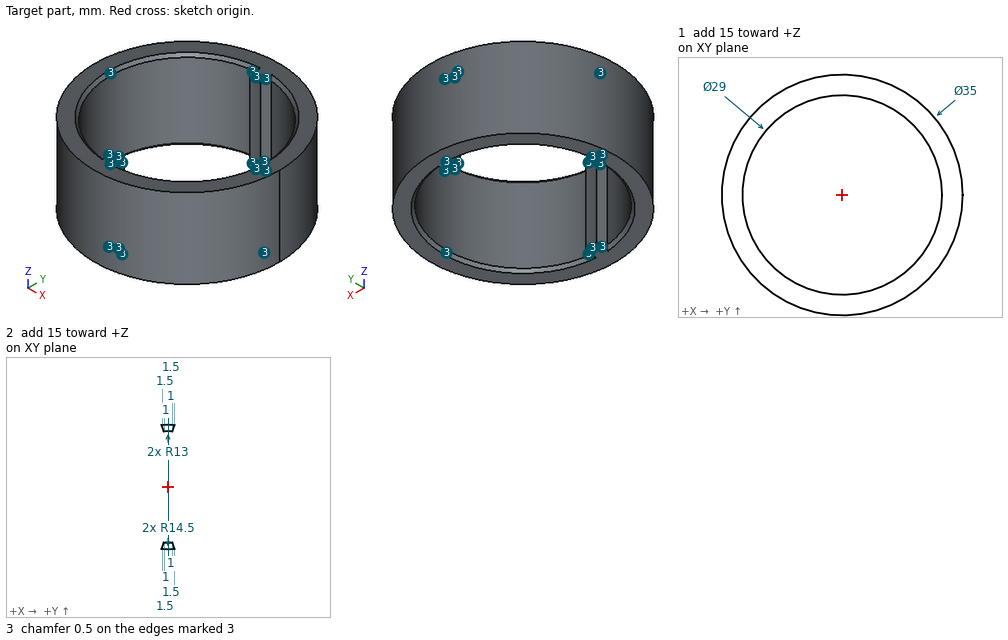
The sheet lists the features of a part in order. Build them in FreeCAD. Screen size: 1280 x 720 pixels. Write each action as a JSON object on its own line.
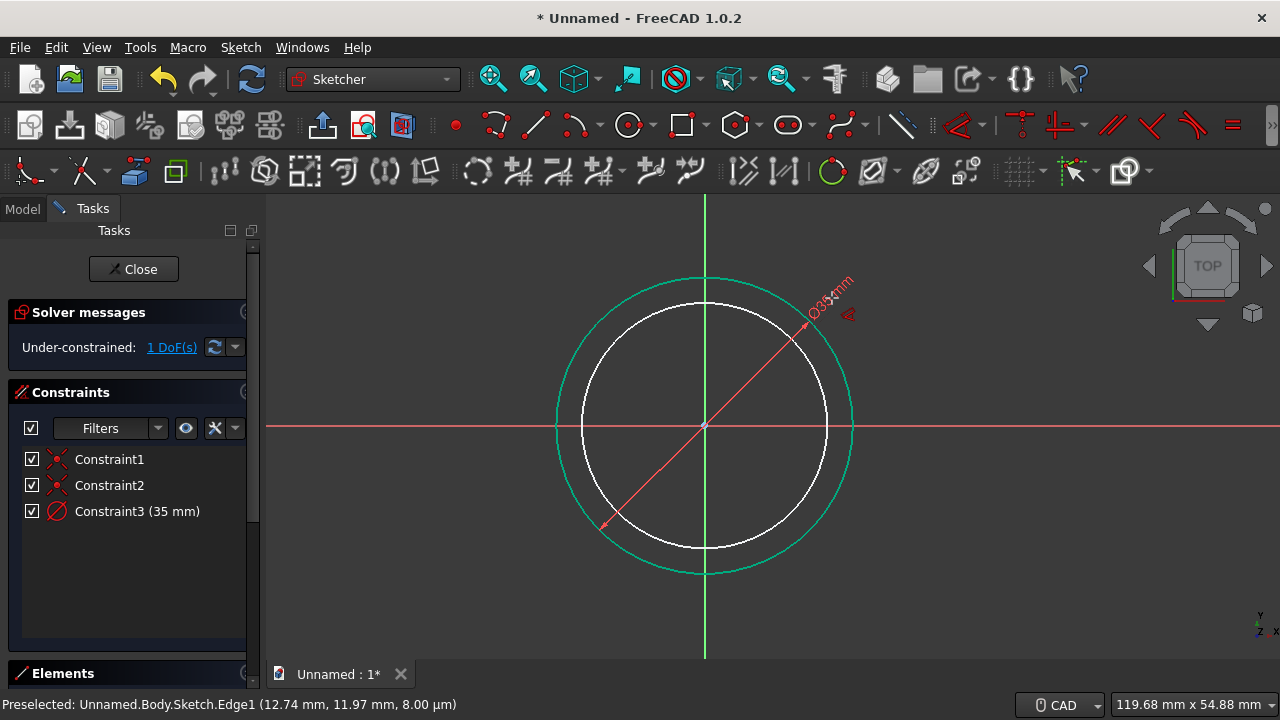
{"action": "left_click", "coordinate": [791, 339]}
{"action": "left_click", "coordinate": [875, 375]}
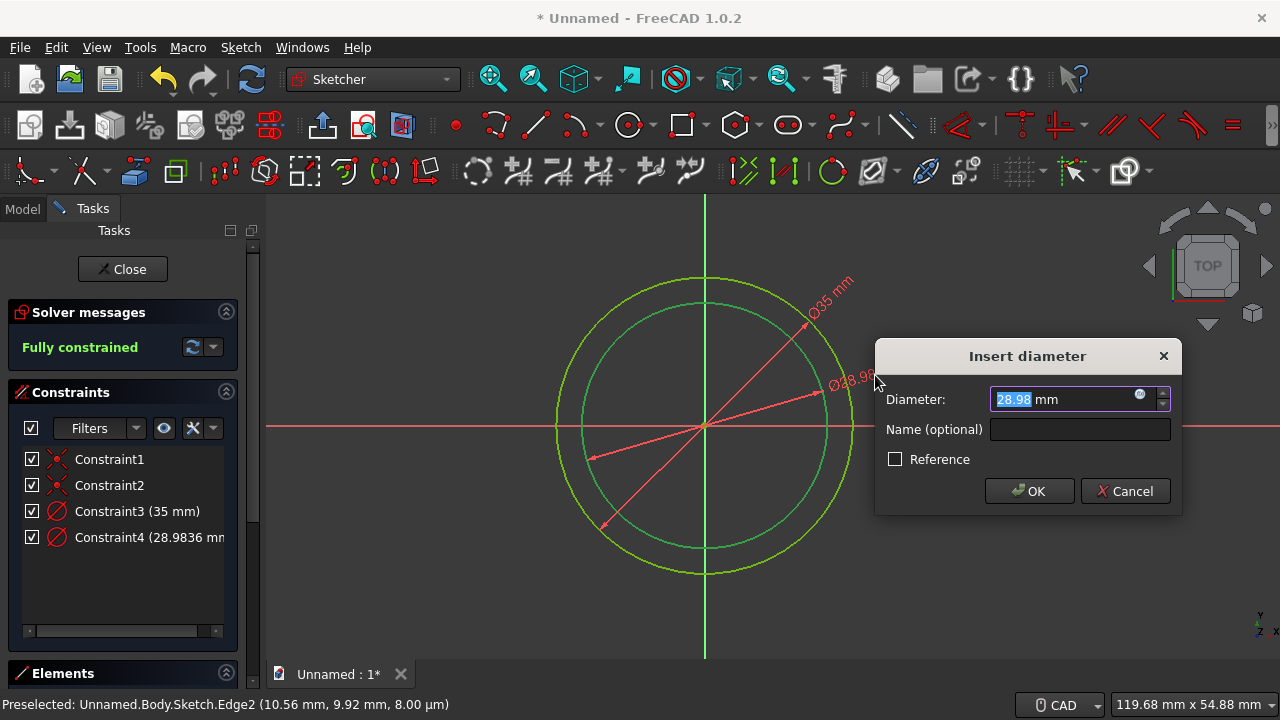
{"action": "type", "text": "29"}
{"action": "key", "text": "Return"}
{"action": "key", "text": "Escape"}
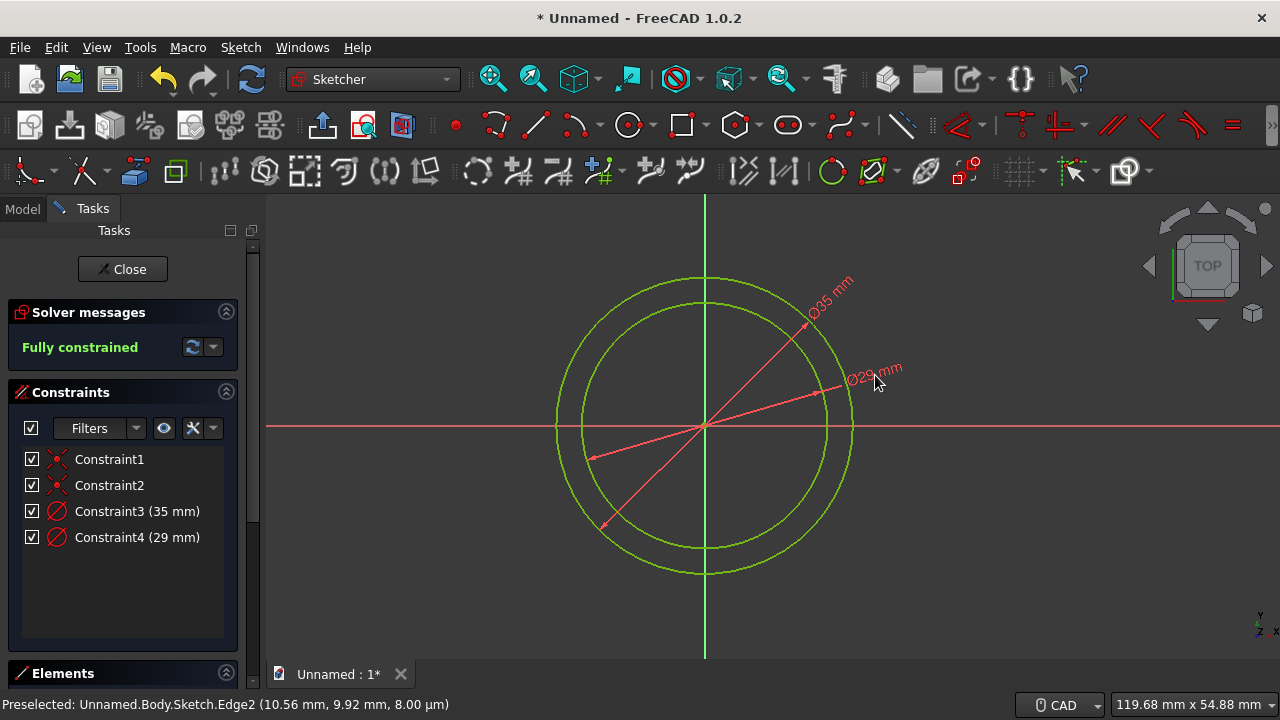
{"action": "left_click", "coordinate": [123, 269]}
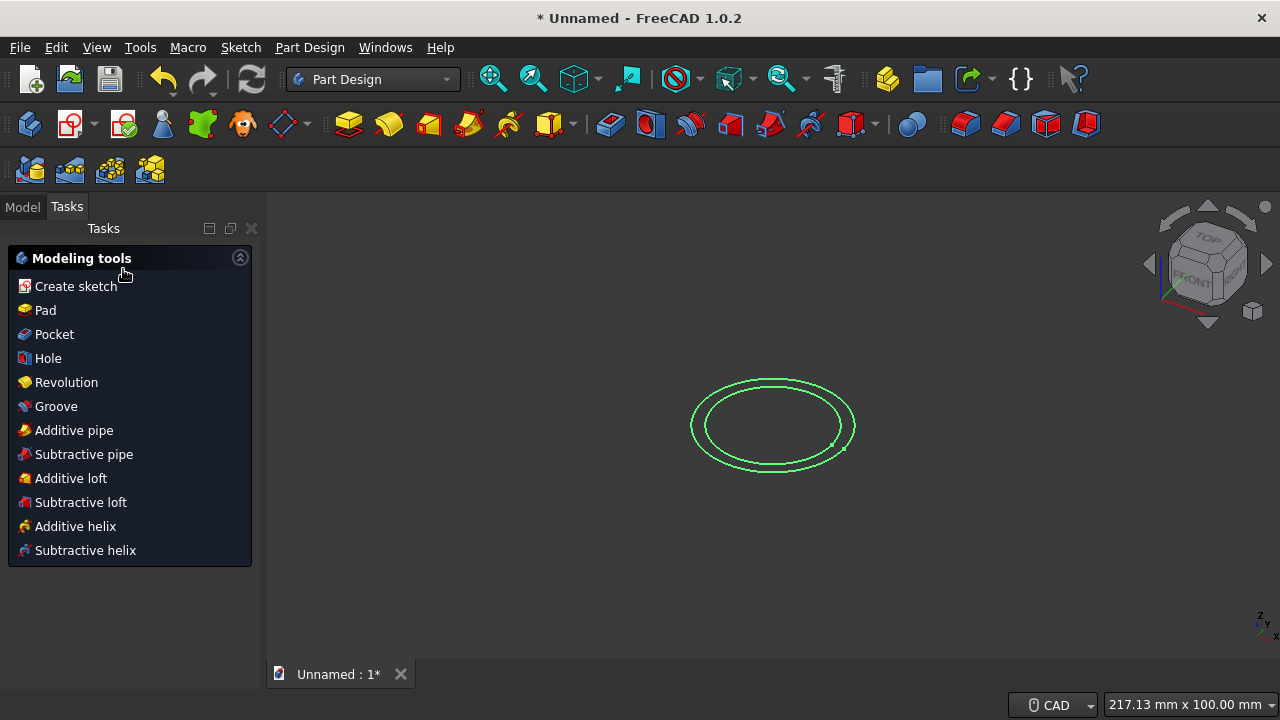
{"action": "left_click", "coordinate": [350, 124]}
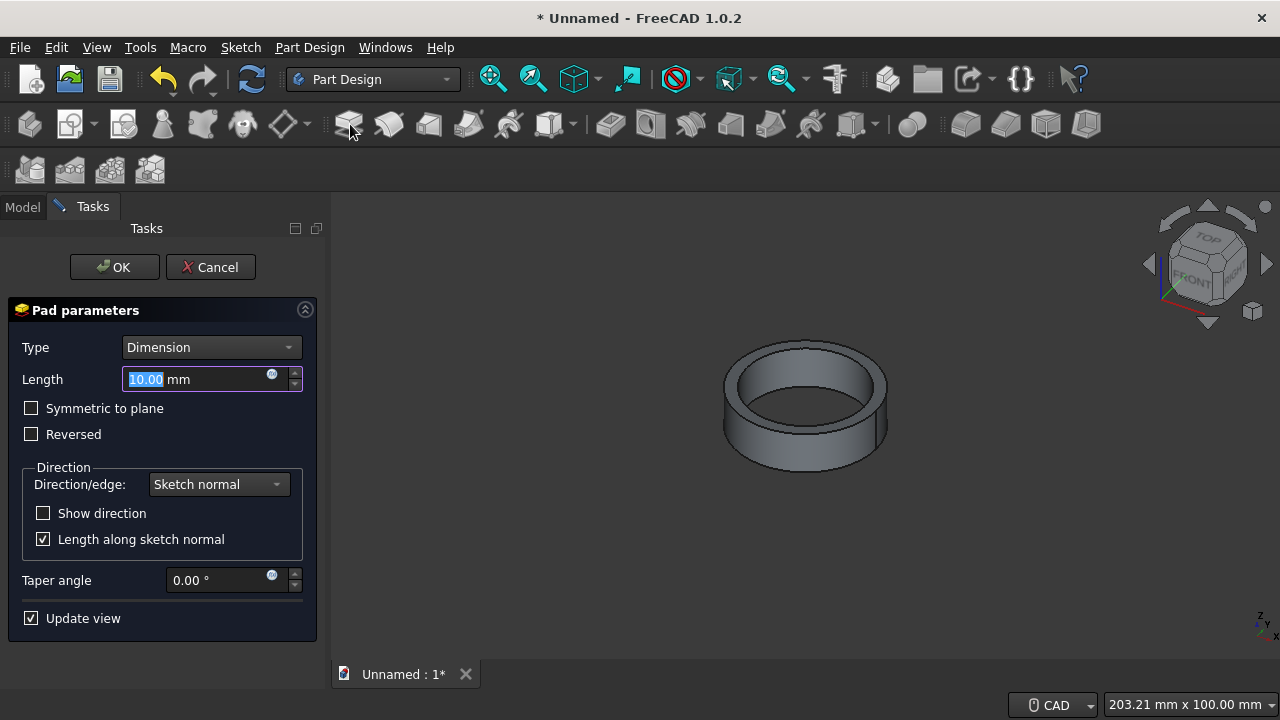
{"action": "type", "text": "15"}
{"action": "key", "text": "Tab"}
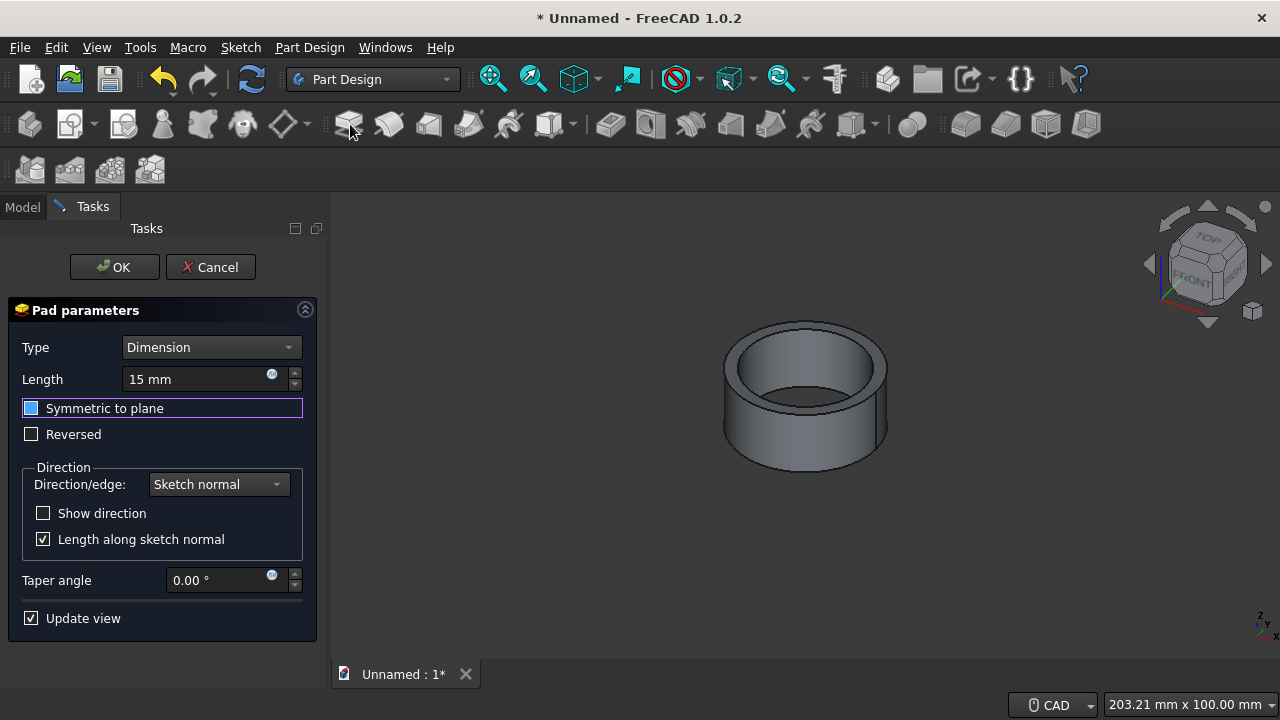
{"action": "left_click", "coordinate": [115, 267]}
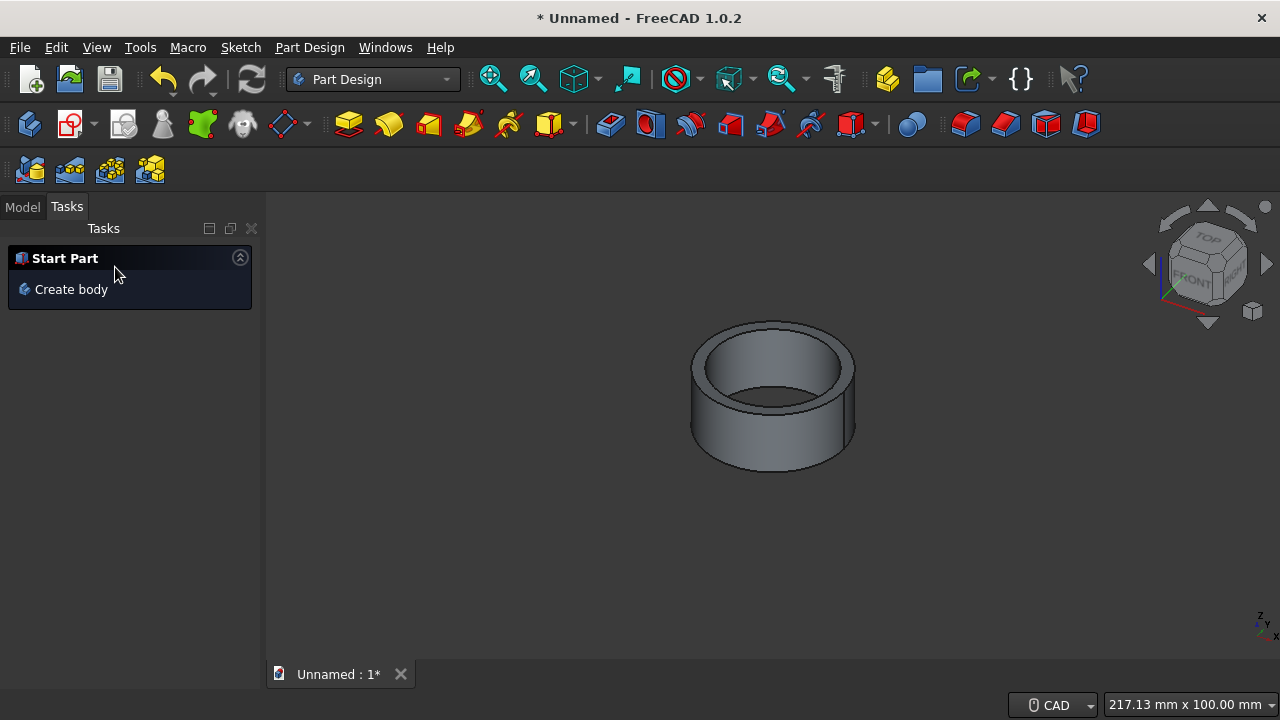
{"action": "key", "text": "v f"}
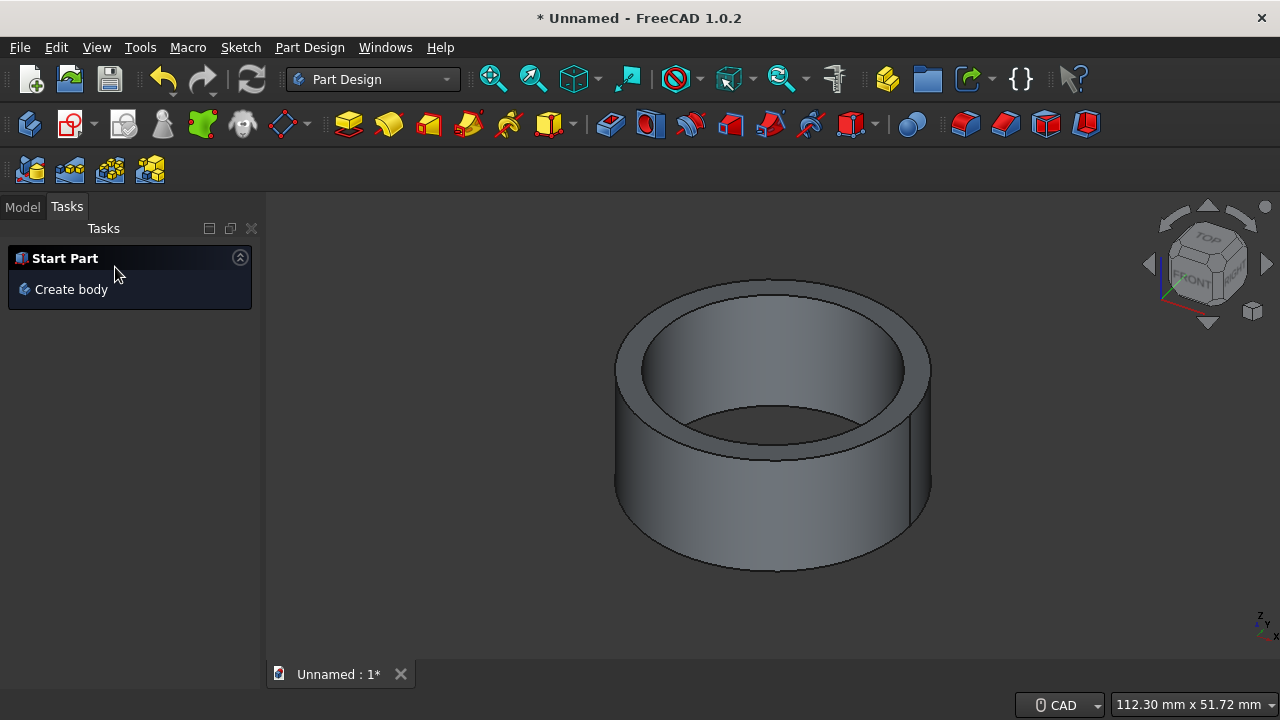
{"action": "left_click", "coordinate": [70, 124]}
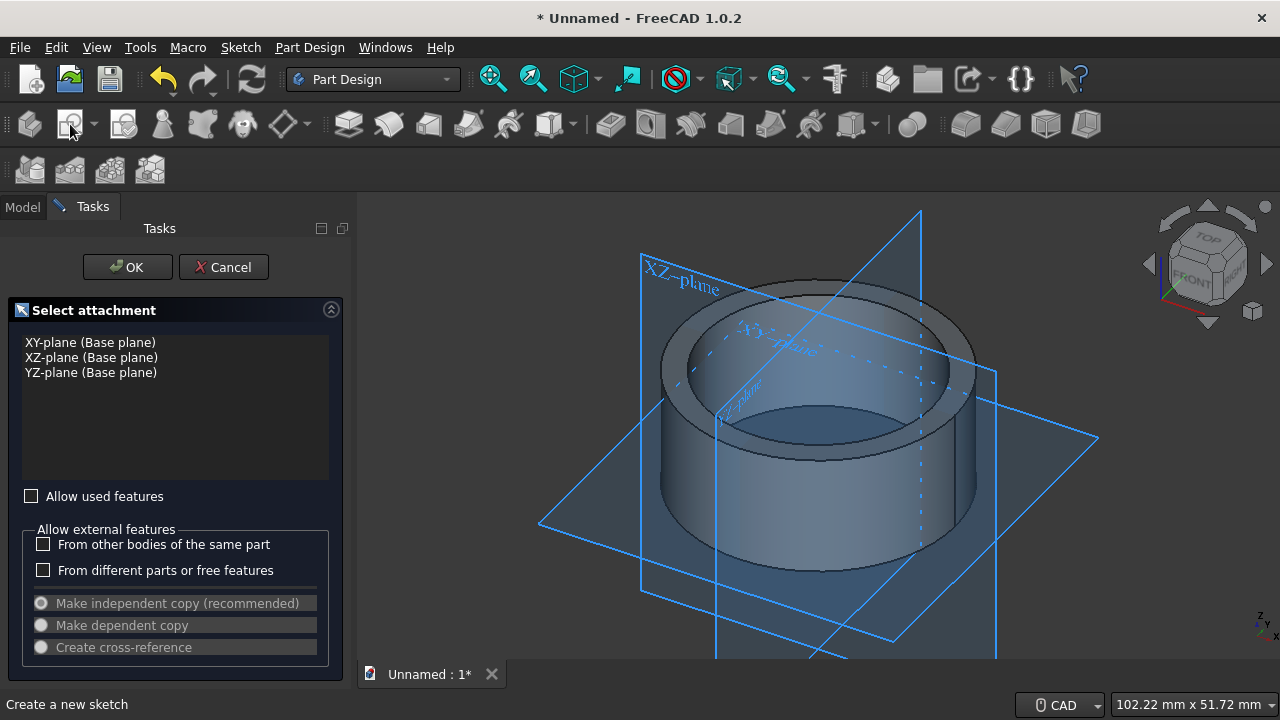
{"action": "left_click", "coordinate": [82, 342]}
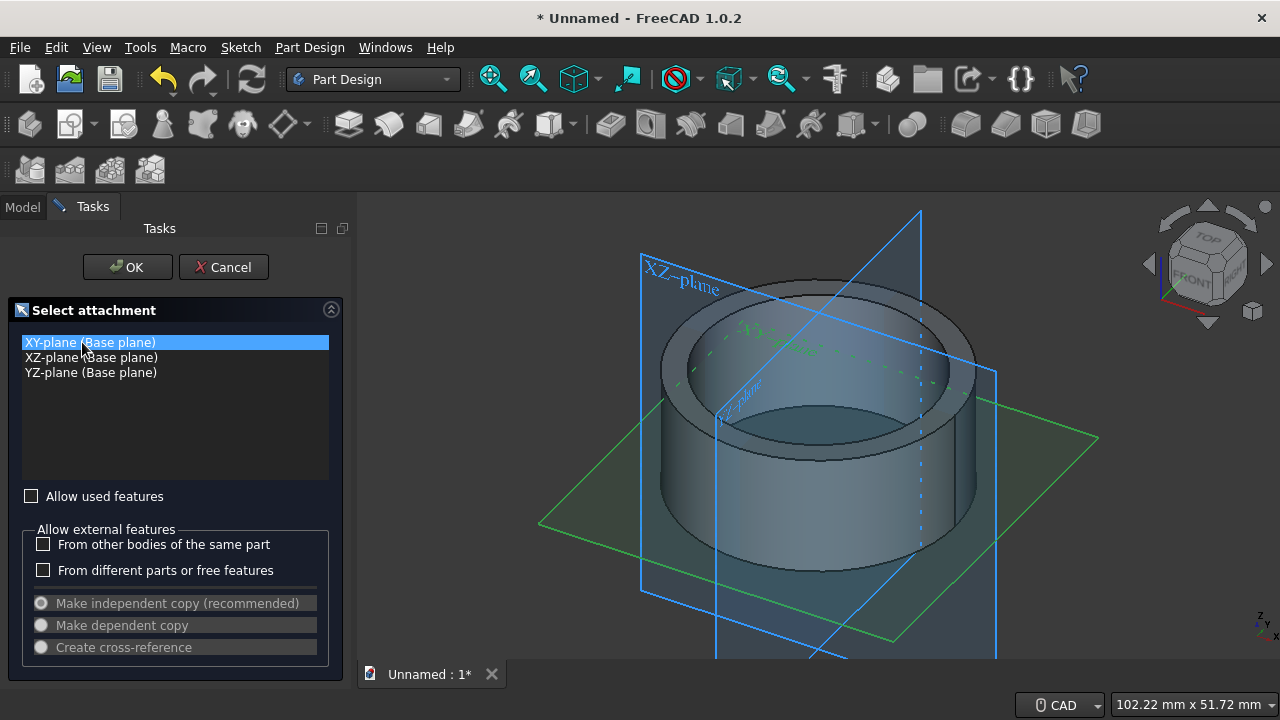
{"action": "left_click", "coordinate": [128, 267]}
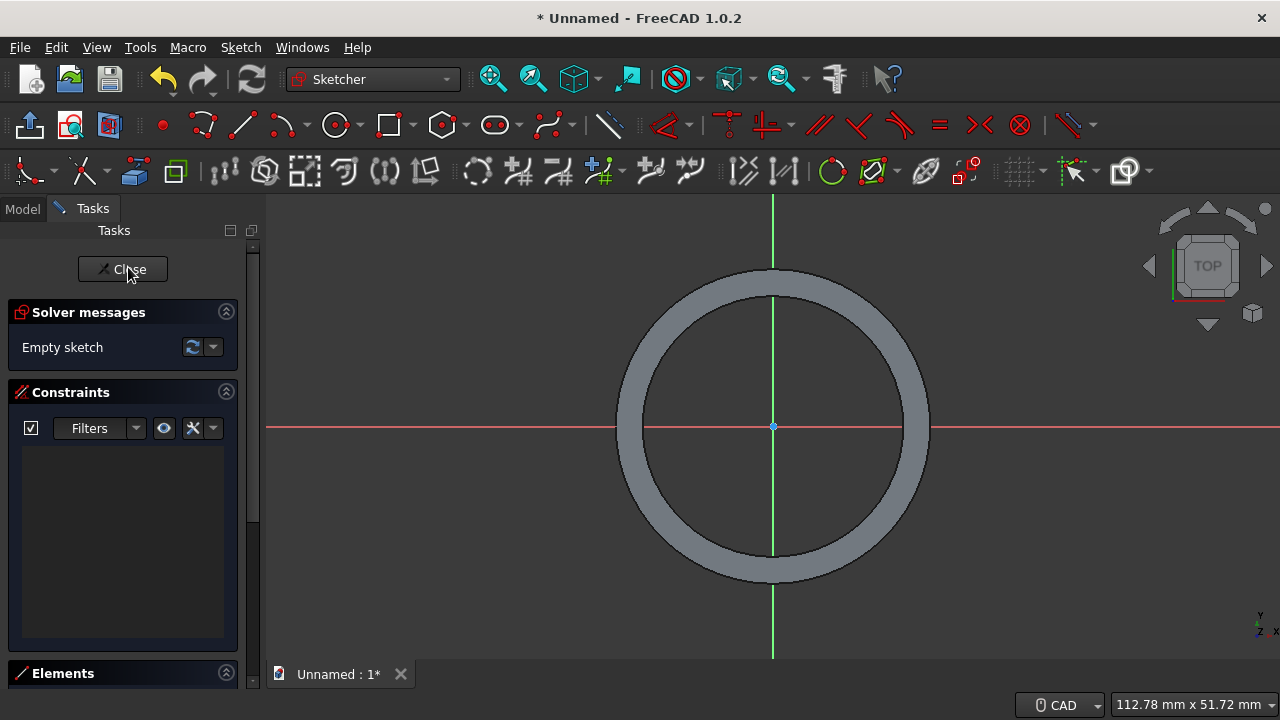
{"action": "left_click", "coordinate": [110, 126]}